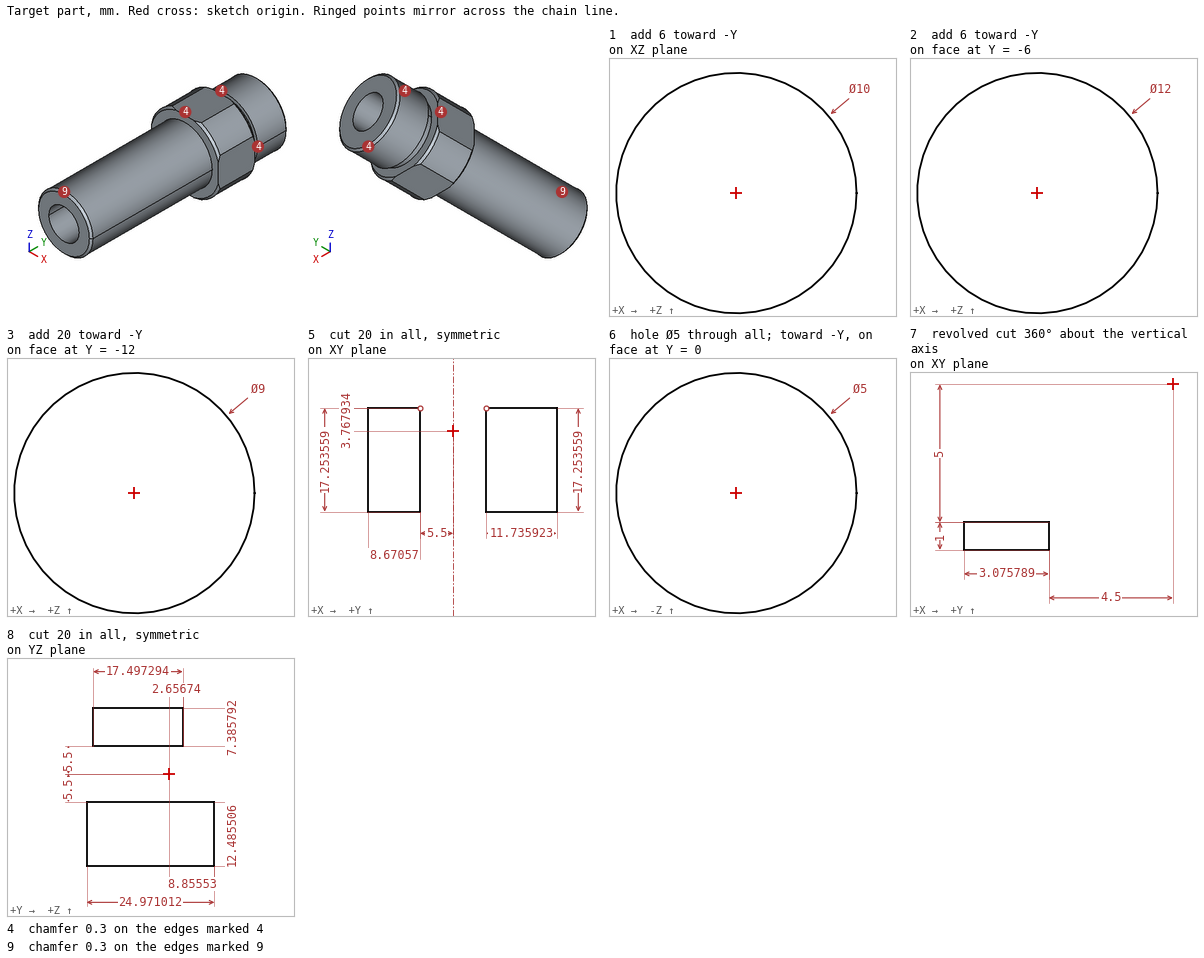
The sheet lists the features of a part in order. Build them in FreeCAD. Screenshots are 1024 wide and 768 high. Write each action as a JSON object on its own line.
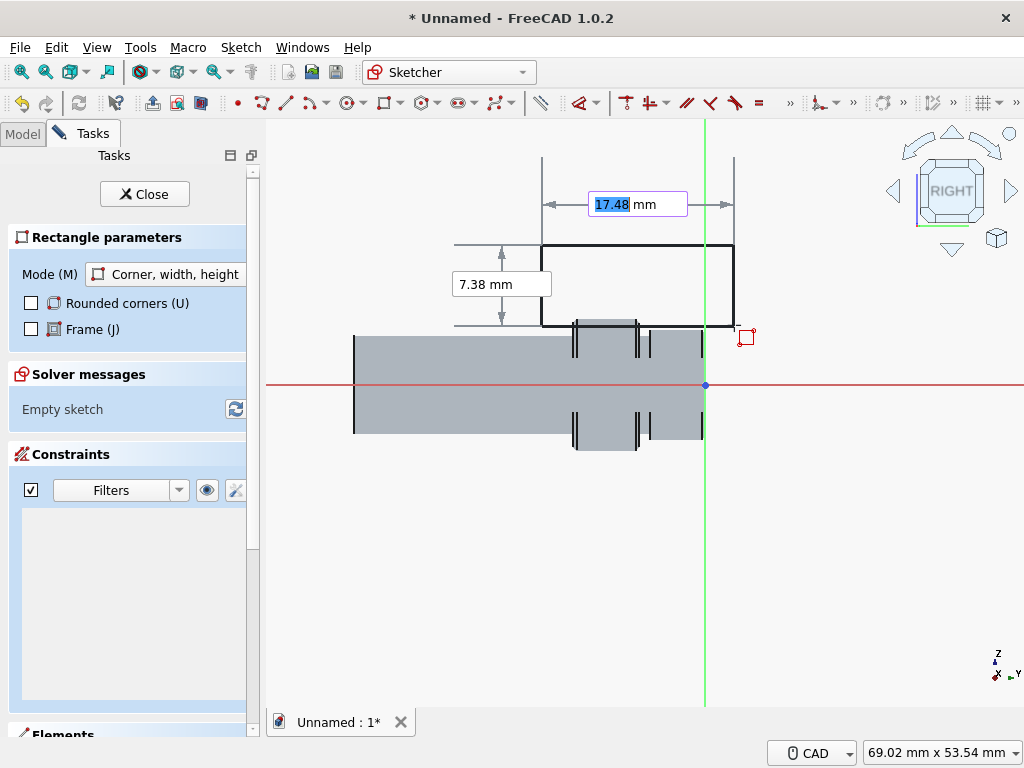
{"action": "type", "text": "17.497294"}
{"action": "key", "text": "Tab"}
{"action": "type", "text": "7.385792"}
{"action": "key", "text": "Return"}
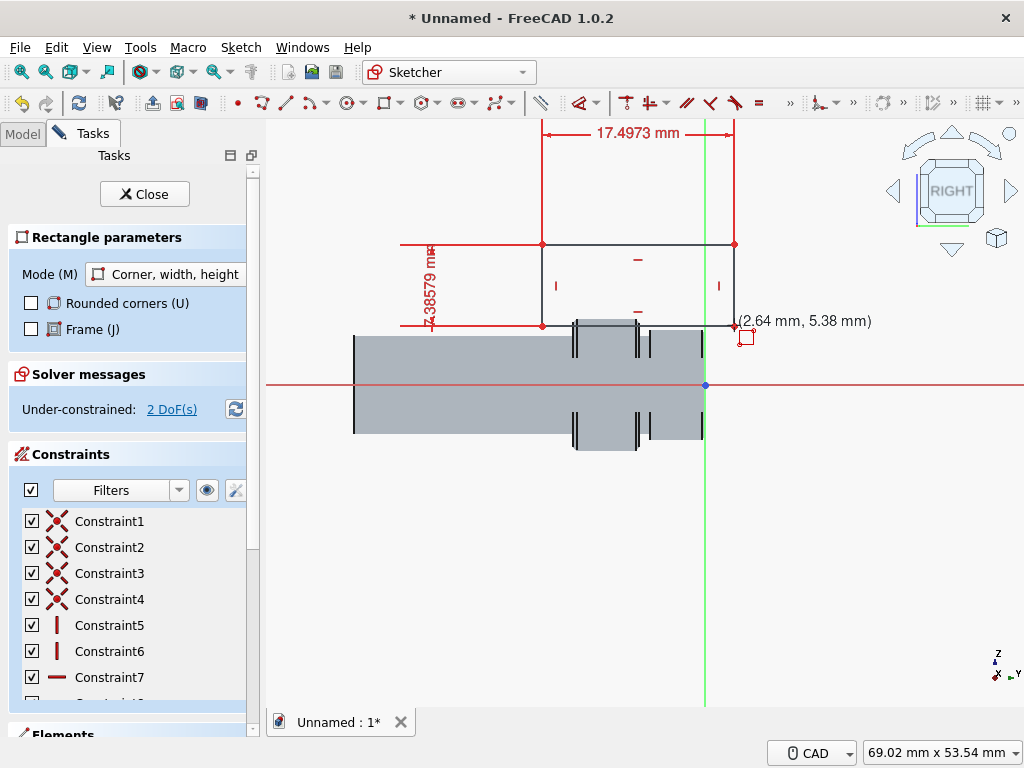
{"action": "left_click", "coordinate": [528, 445]}
{"action": "mouse_move", "coordinate": [802, 583]}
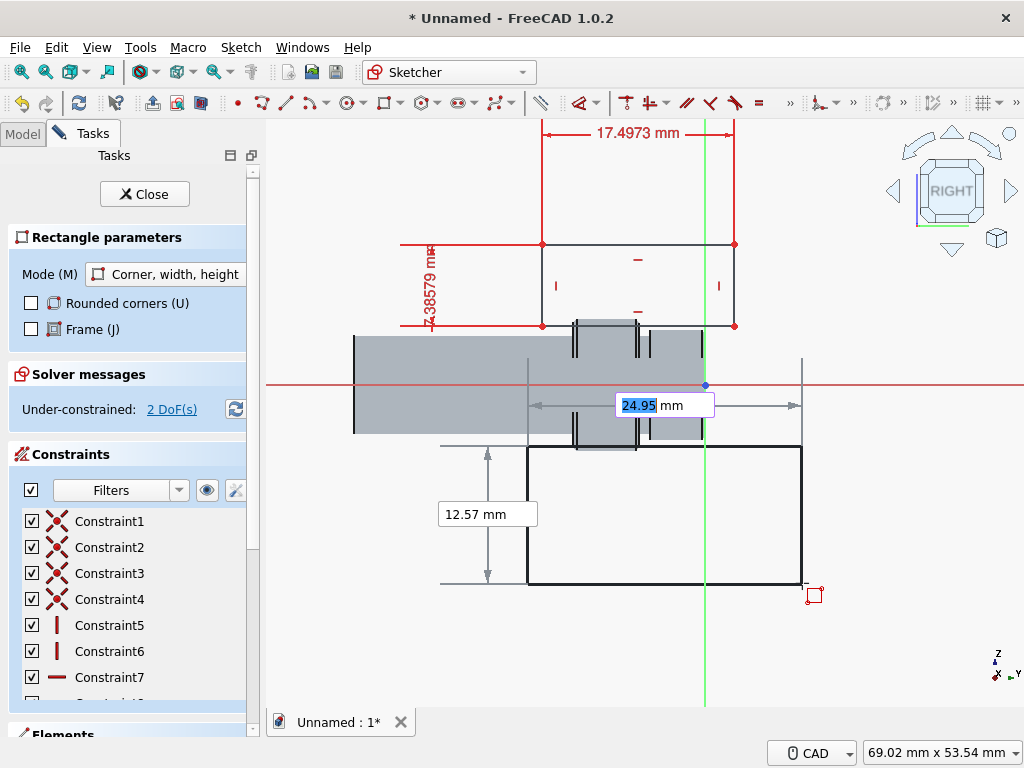
{"action": "type", "text": "24.971012"}
{"action": "key", "text": "Tab"}
{"action": "type", "text": "12.485506"}
{"action": "key", "text": "Return"}
{"action": "key", "text": "Escape"}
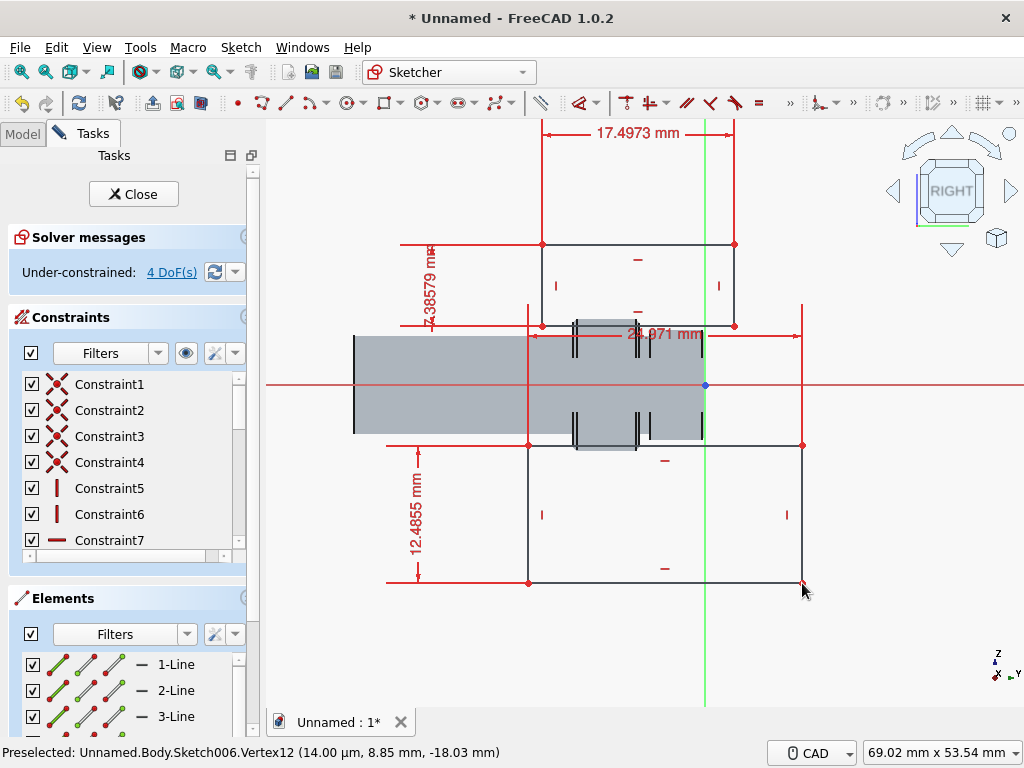
{"action": "left_click", "coordinate": [580, 104]}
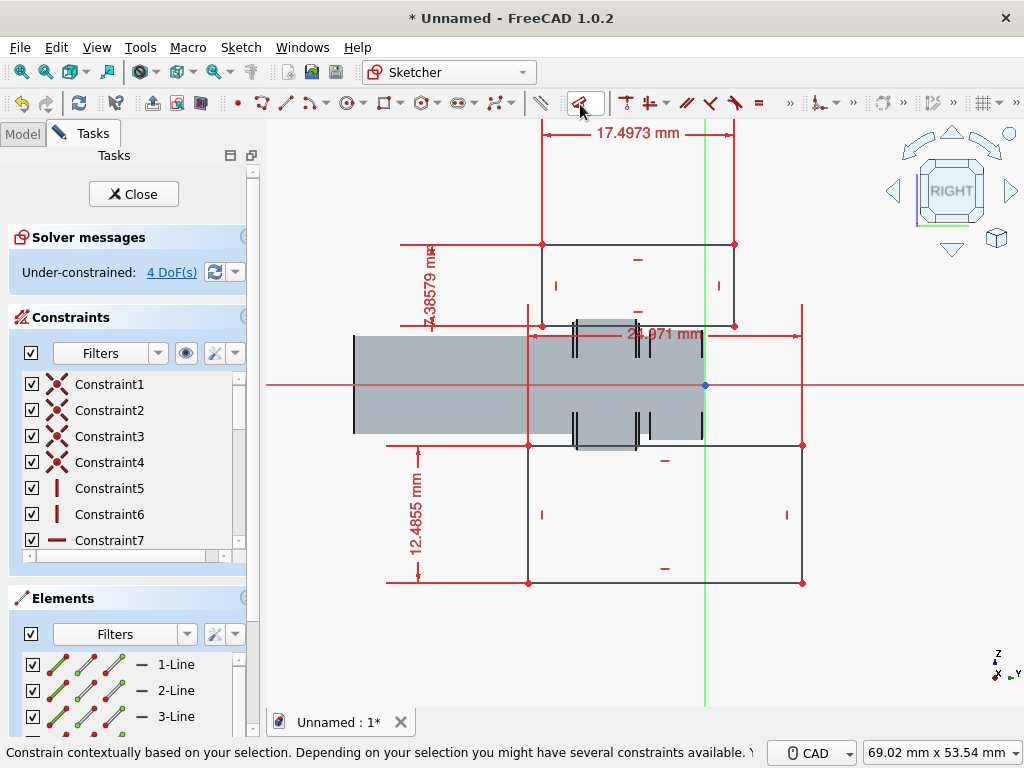
{"action": "left_click", "coordinate": [542, 326]}
{"action": "left_click", "coordinate": [508, 356]}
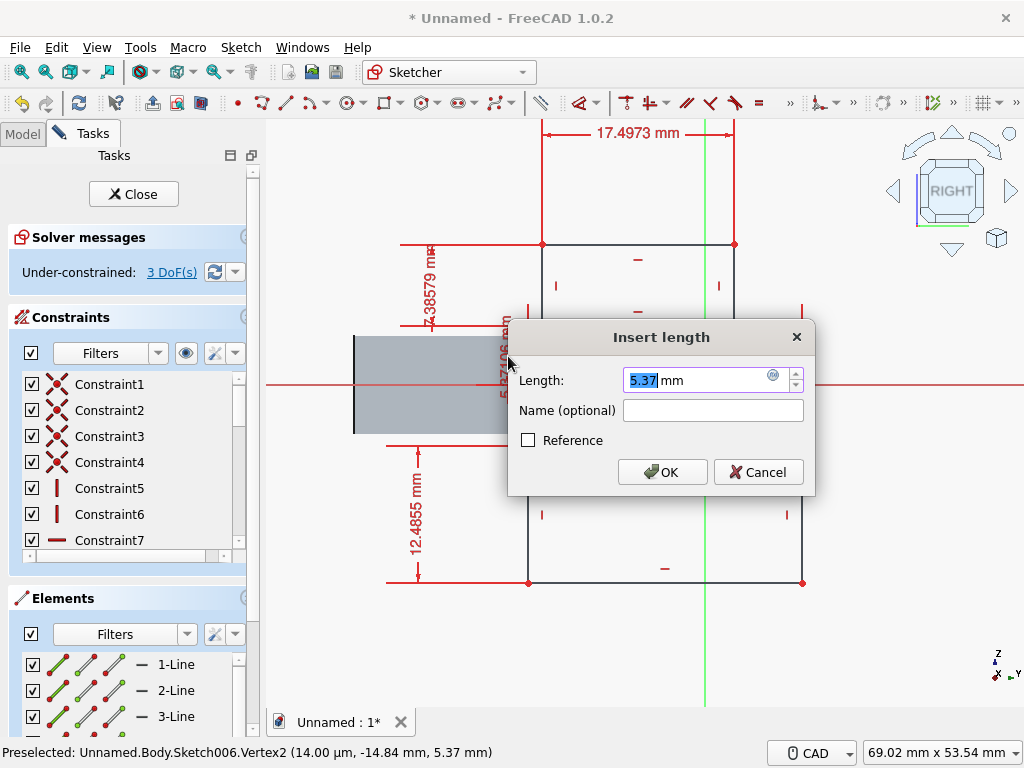
{"action": "type", "text": "5.5"}
{"action": "key", "text": "Return"}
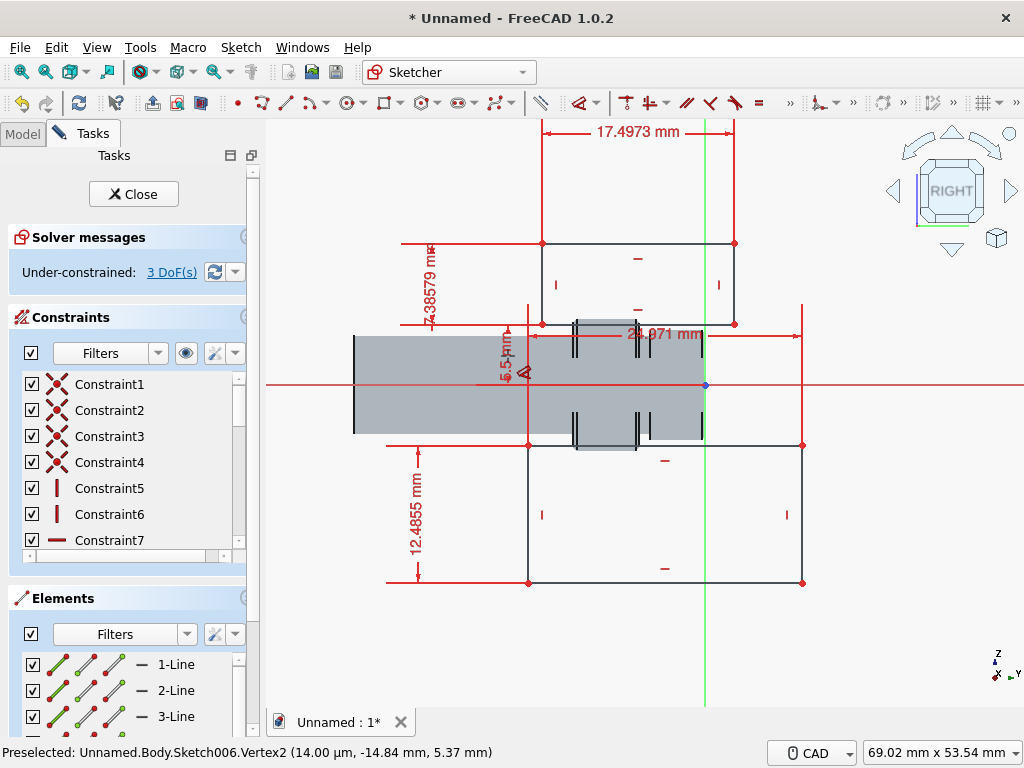
{"action": "left_click", "coordinate": [528, 446]}
{"action": "left_click", "coordinate": [494, 416]}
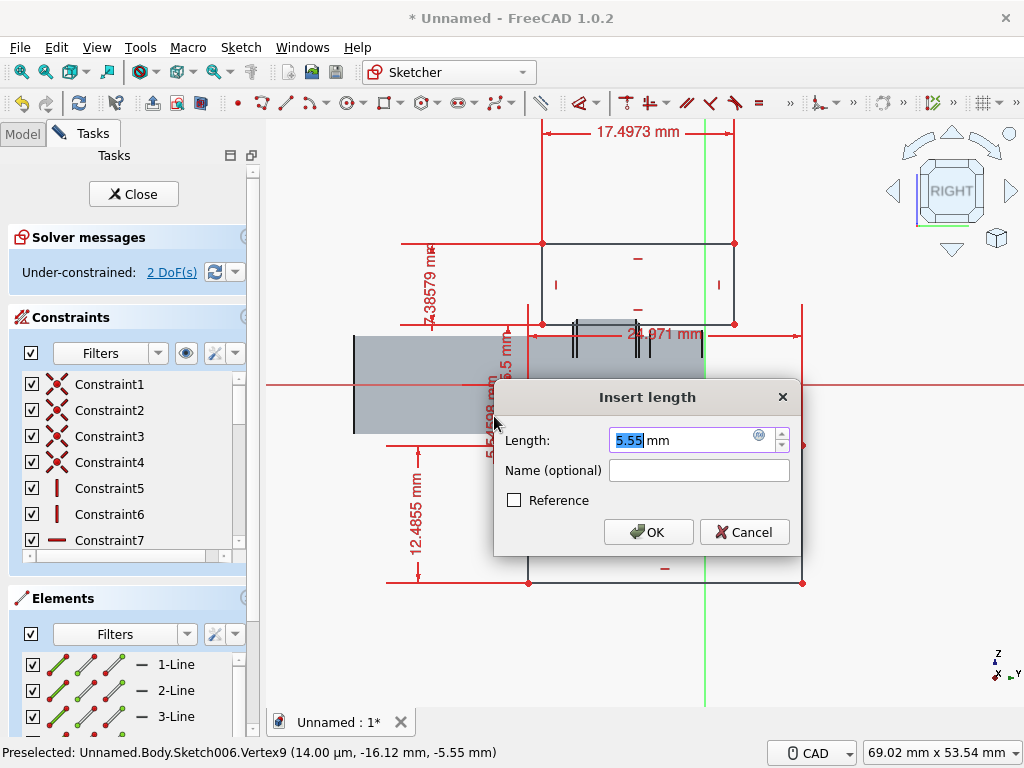
{"action": "type", "text": "5.5"}
{"action": "key", "text": "Return"}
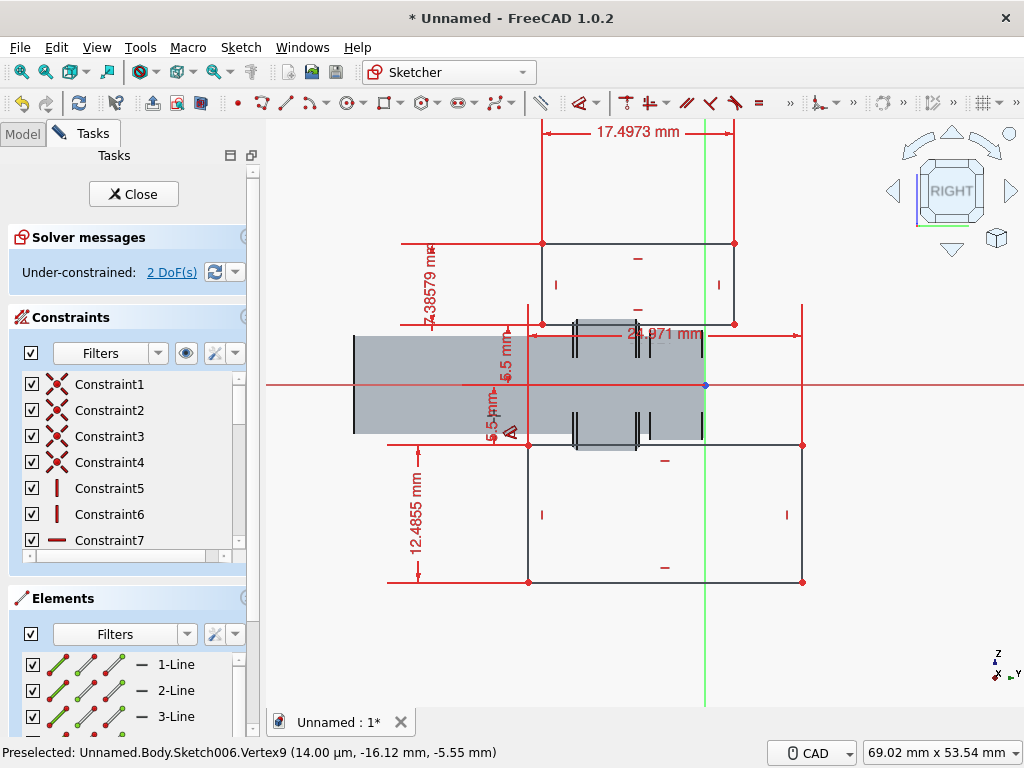
{"action": "scroll", "coordinate": [734, 325], "scroll_direction": "up", "scroll_amount": 2}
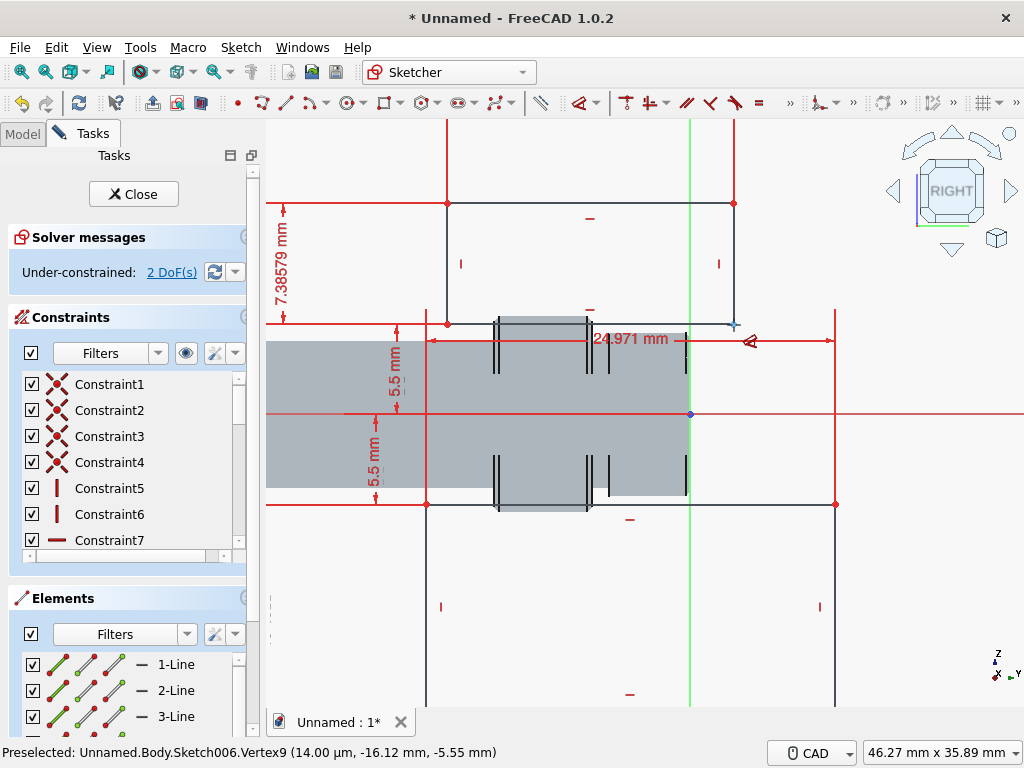
{"action": "left_click", "coordinate": [734, 324]}
{"action": "left_click", "coordinate": [712, 290]}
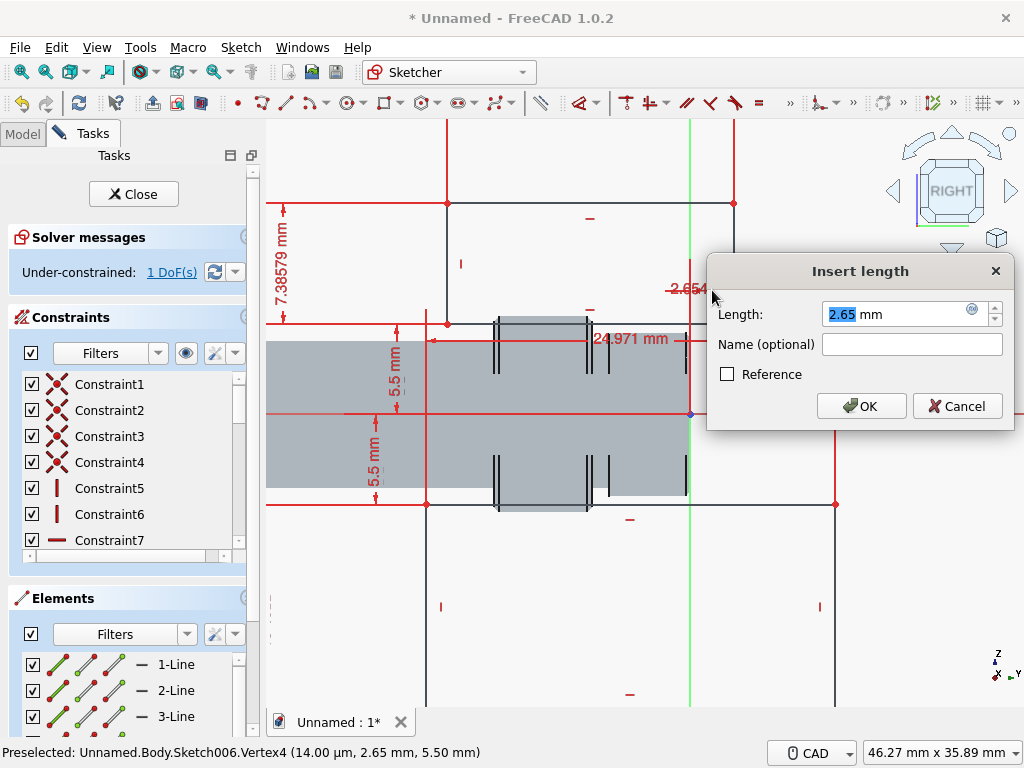
{"action": "type", "text": "2.65674"}
{"action": "key", "text": "Return"}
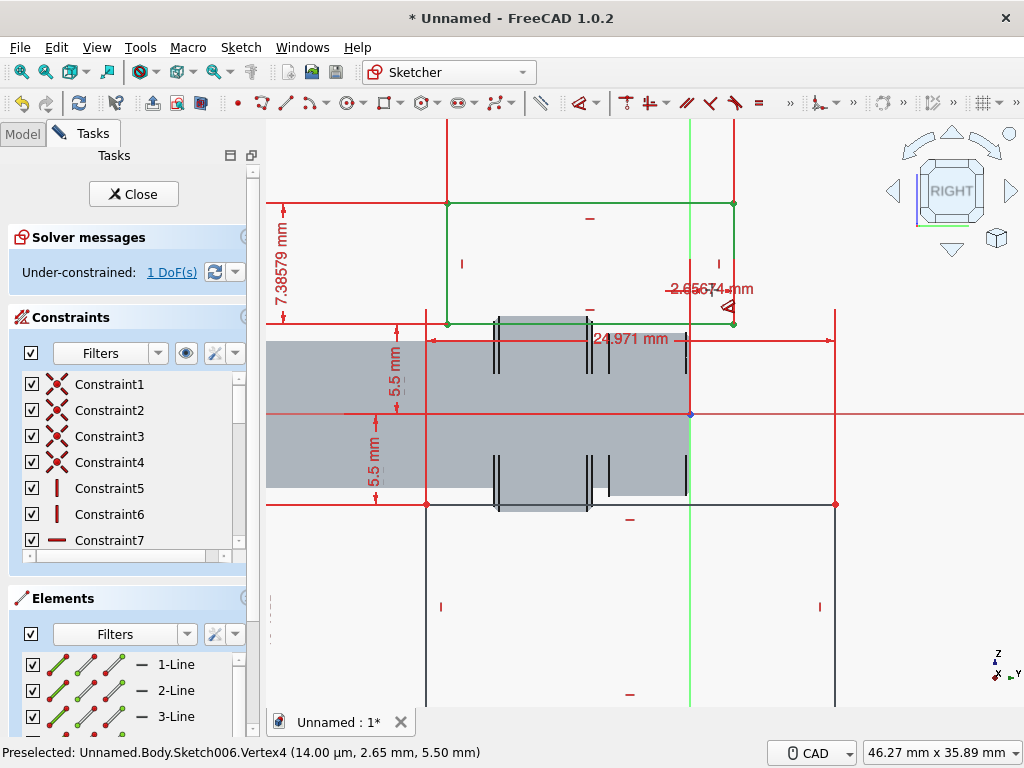
{"action": "scroll", "coordinate": [330, 218], "scroll_direction": "down", "scroll_amount": 1}